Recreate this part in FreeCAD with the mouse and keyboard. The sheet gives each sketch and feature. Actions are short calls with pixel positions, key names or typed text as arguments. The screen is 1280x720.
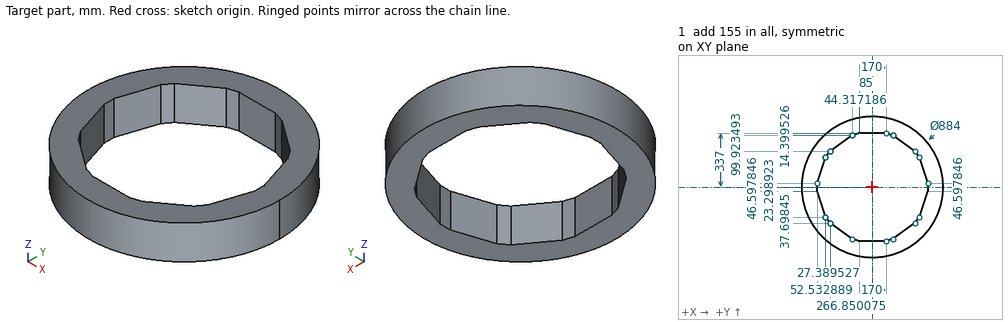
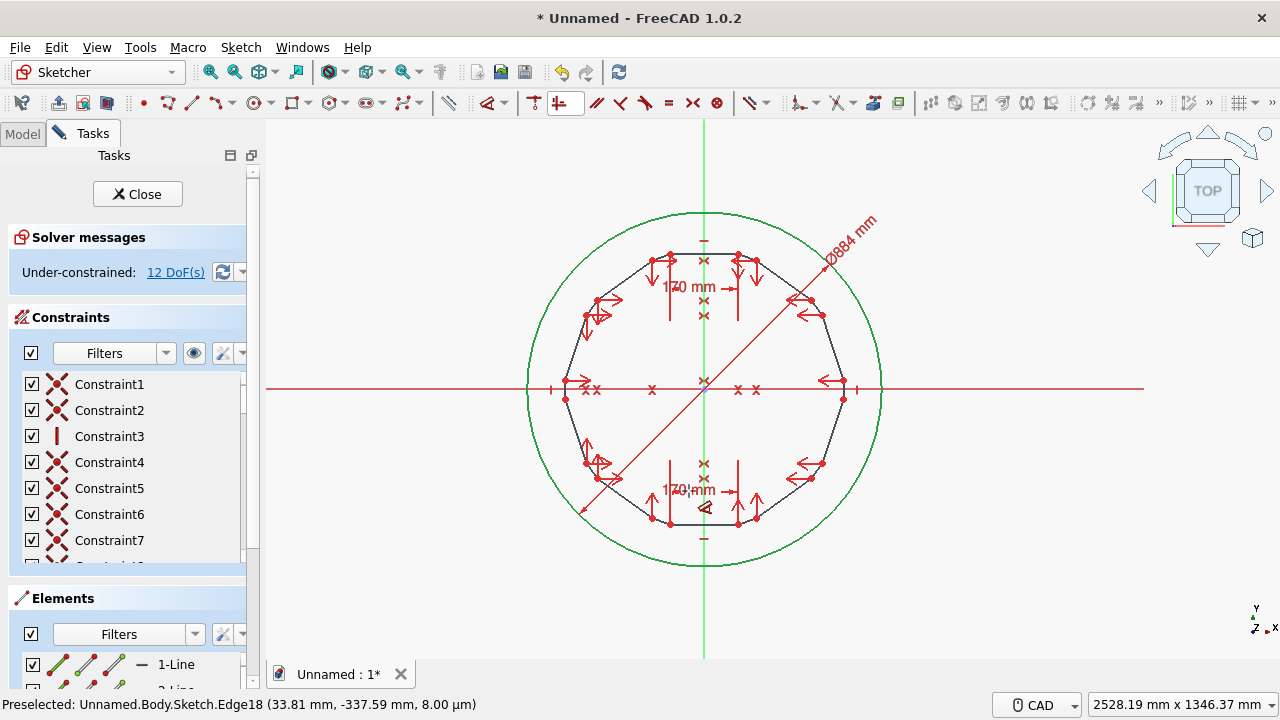
click(670, 254)
click(687, 423)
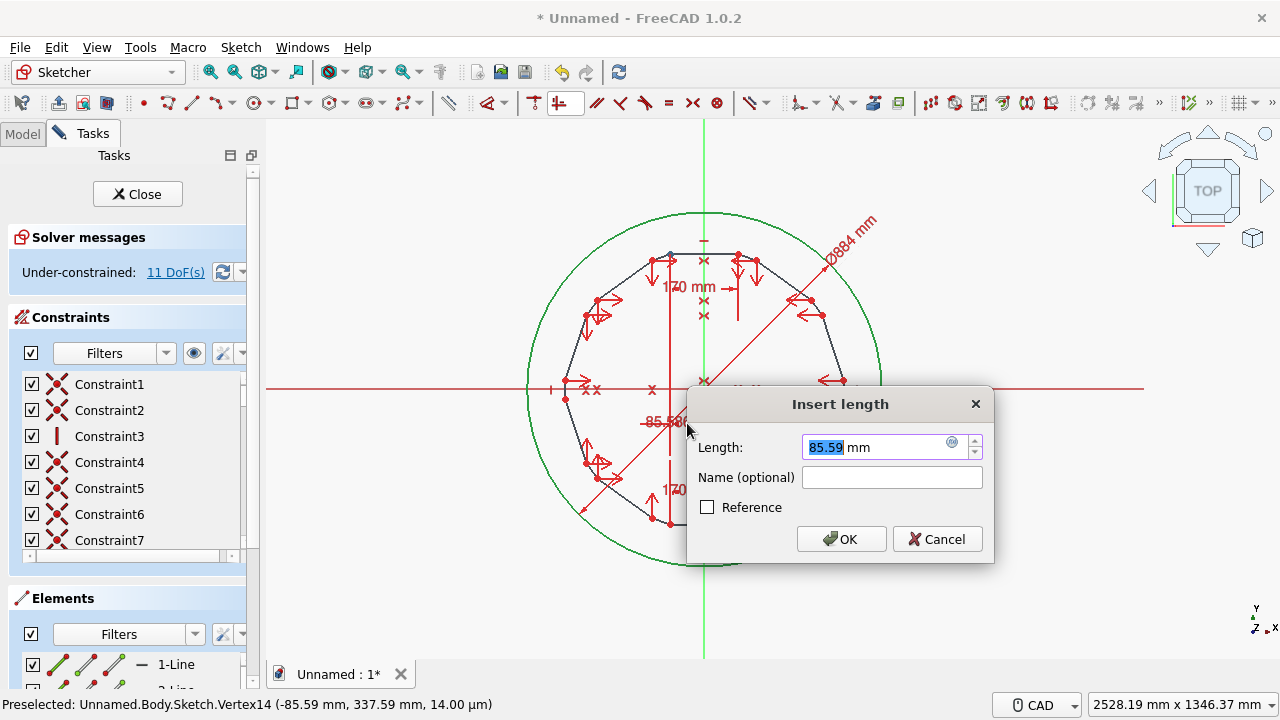
text(85)
key(Return)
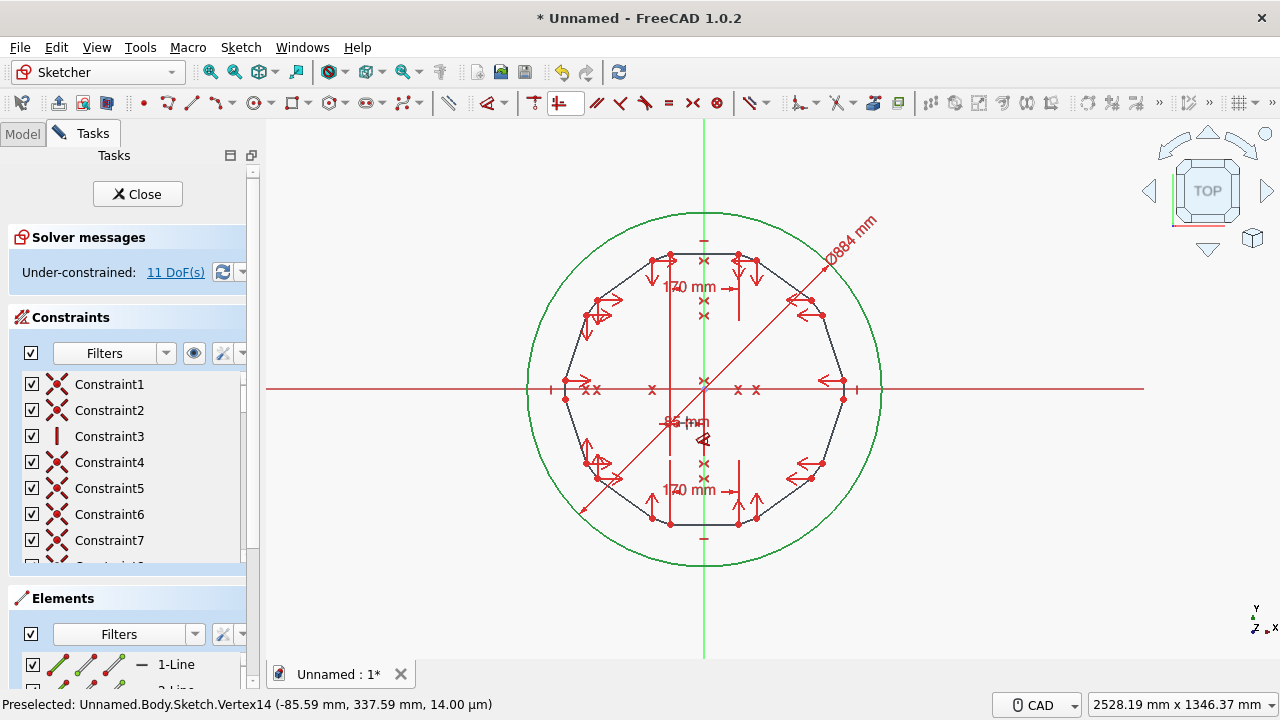
click(670, 254)
click(636, 322)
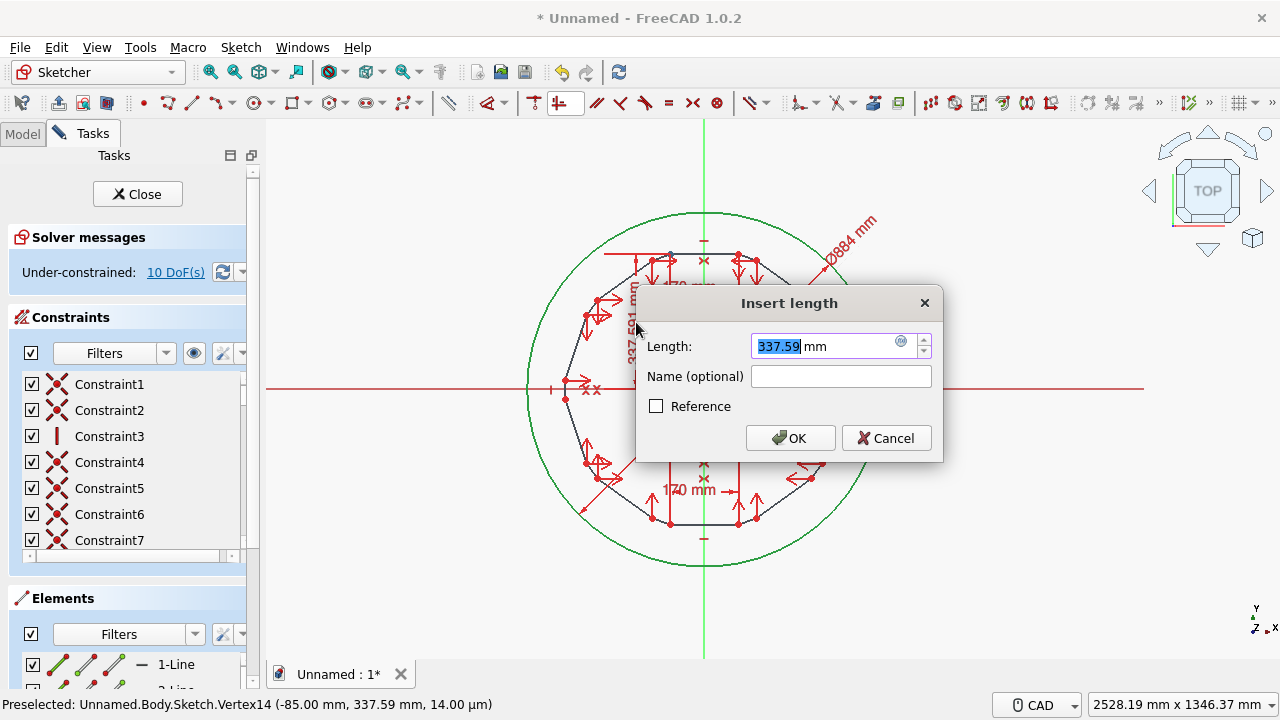
text(337)
key(Return)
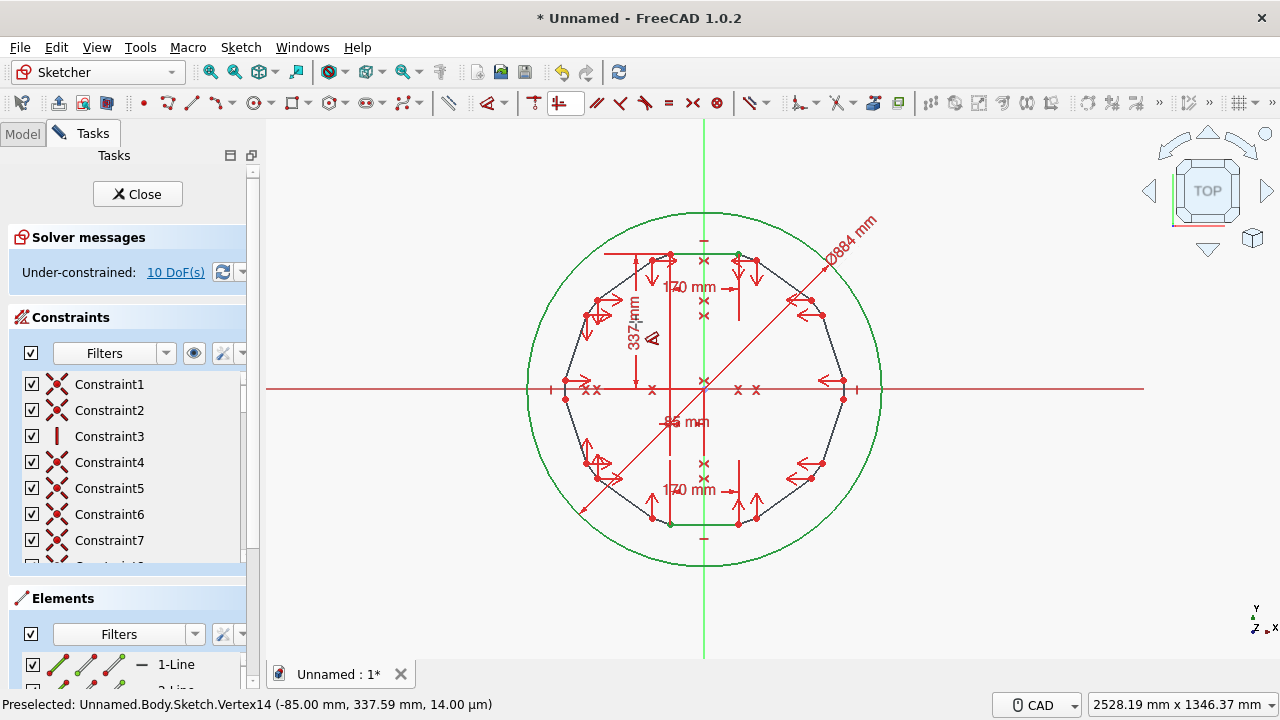
scroll(565, 390, up, 4)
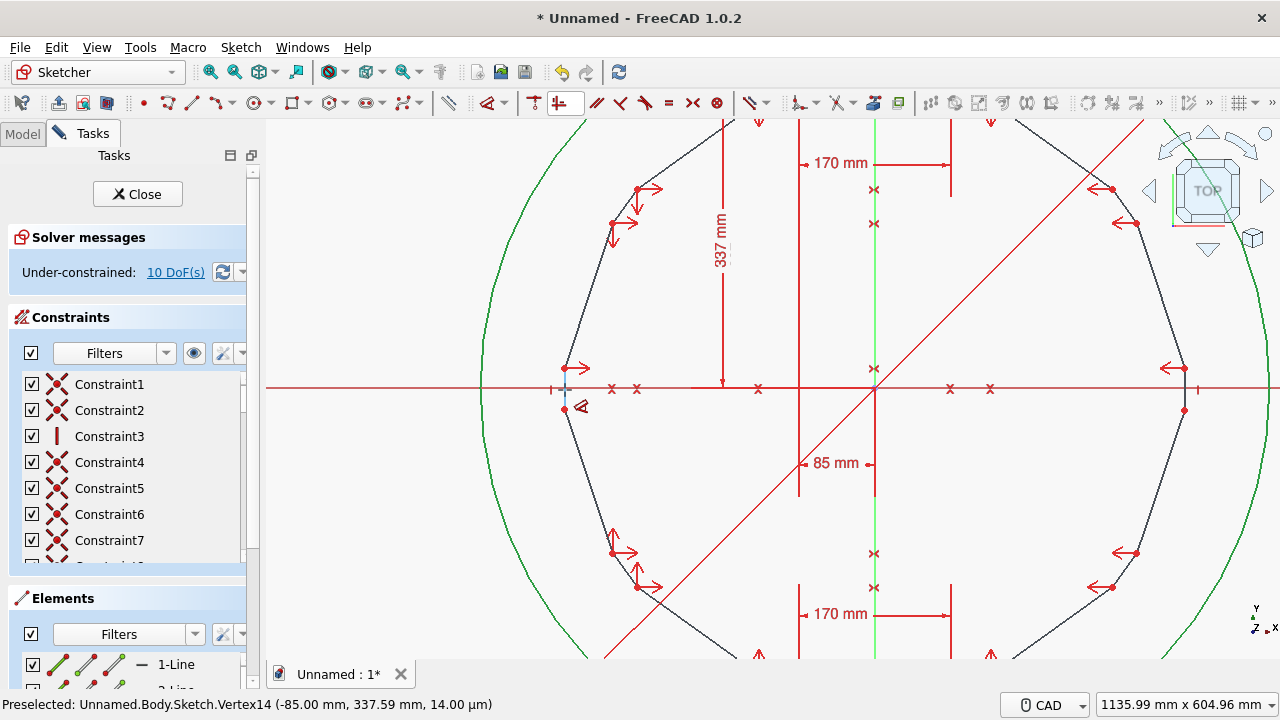
click(565, 389)
click(531, 375)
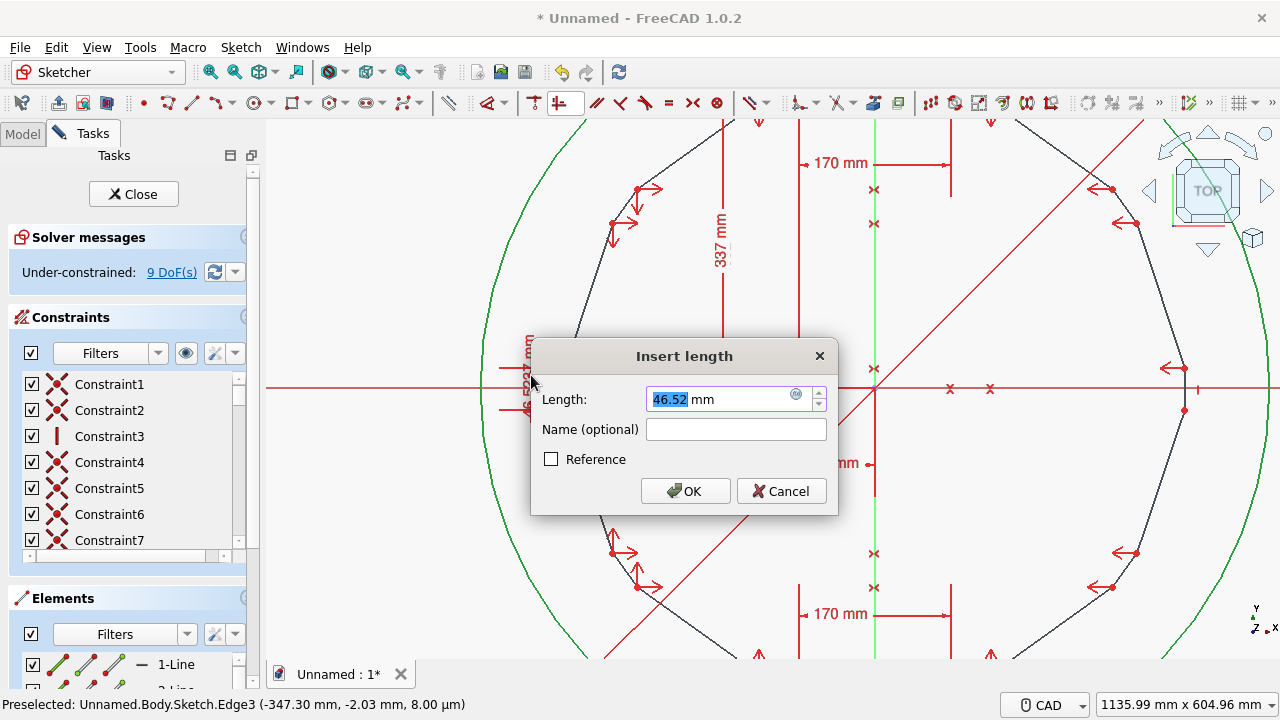
text(46.597846)
key(Return)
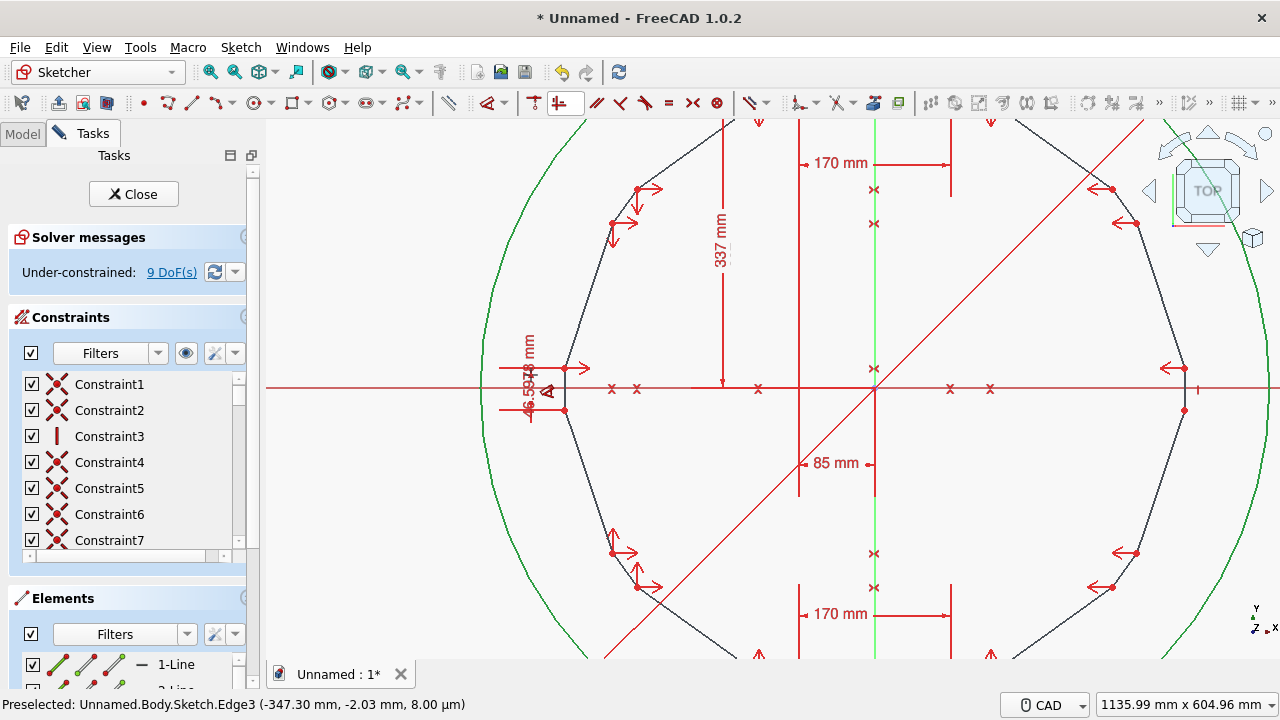
scroll(565, 390, down, 4)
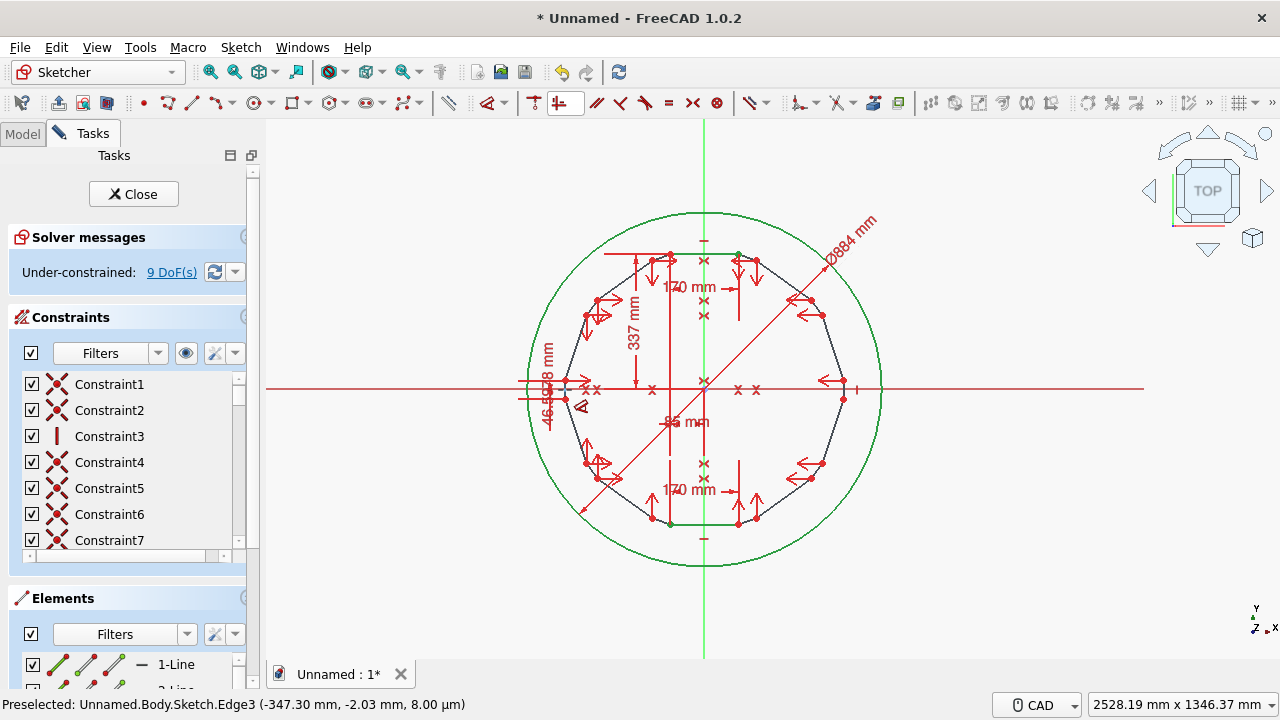
scroll(844, 394, up, 6)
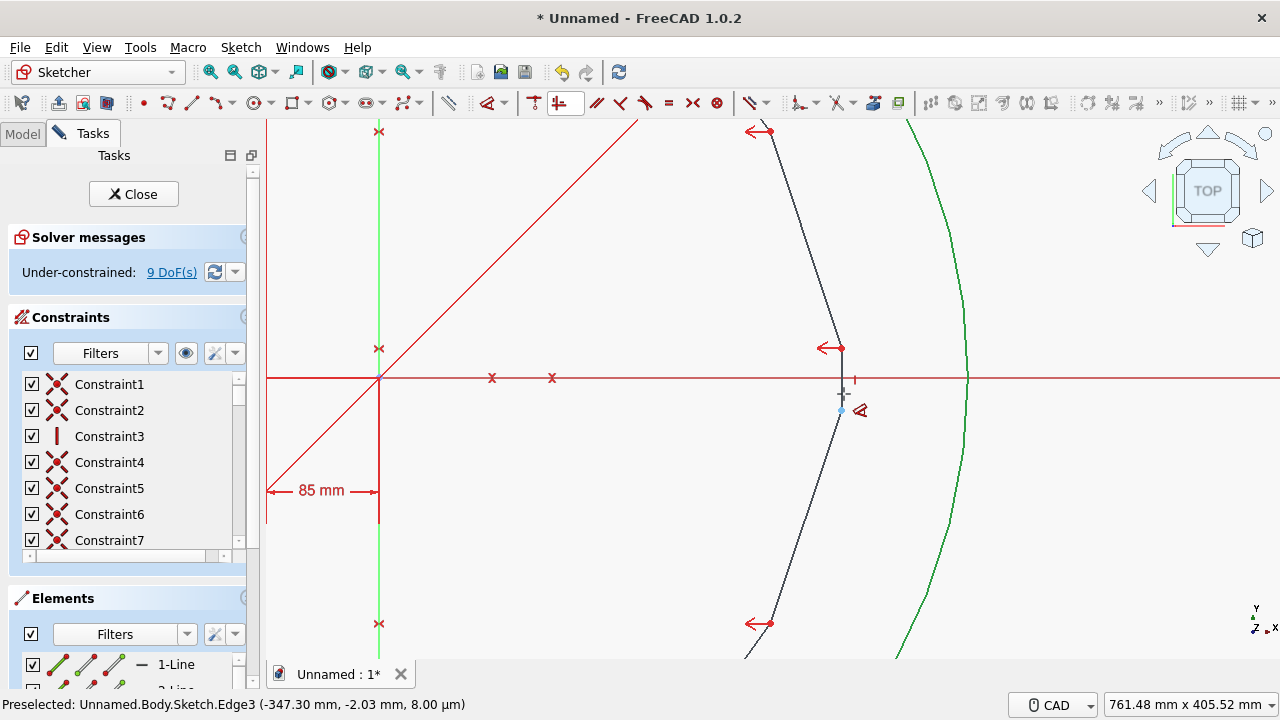
click(842, 392)
click(876, 394)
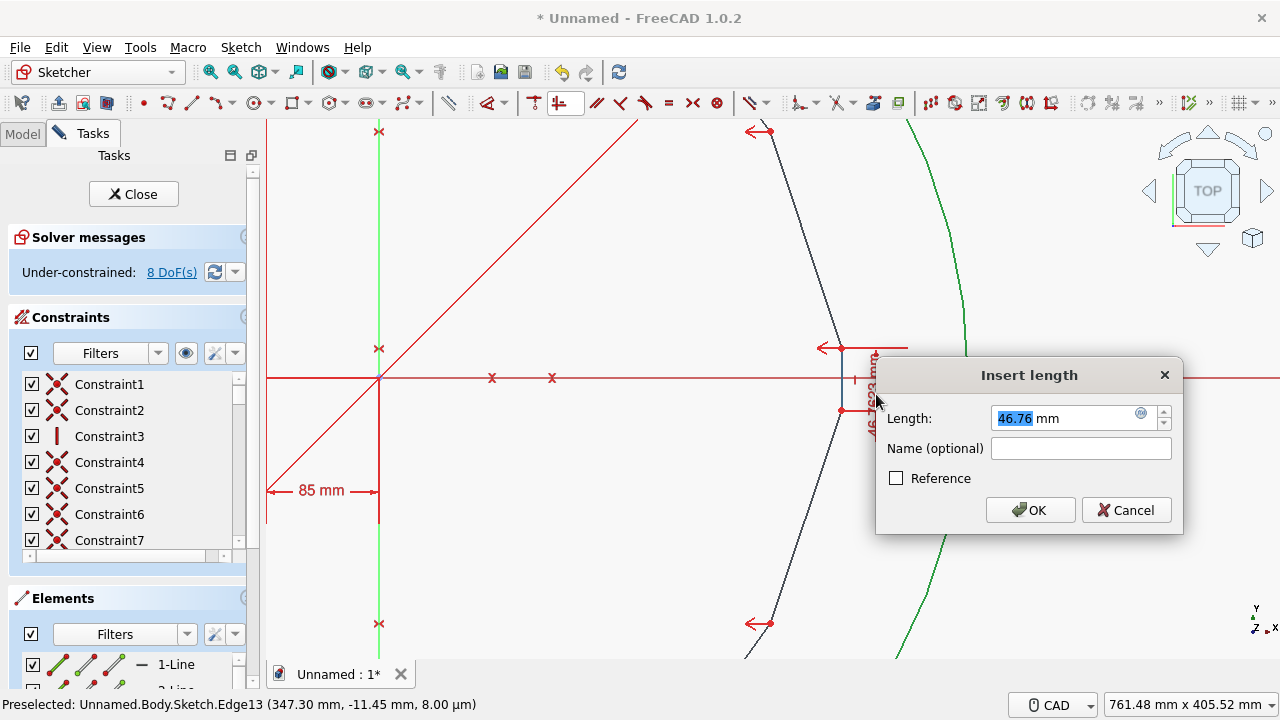
text(46.597846)
key(Return)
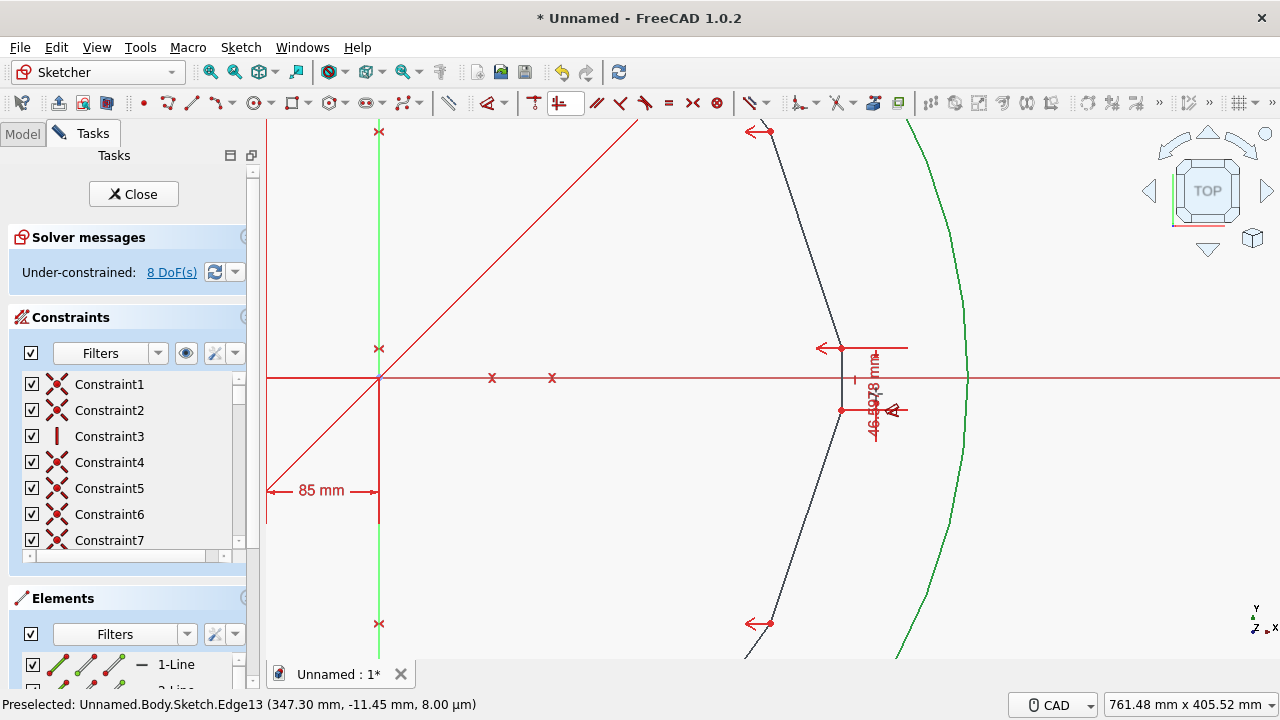
scroll(845, 394, down, 6)